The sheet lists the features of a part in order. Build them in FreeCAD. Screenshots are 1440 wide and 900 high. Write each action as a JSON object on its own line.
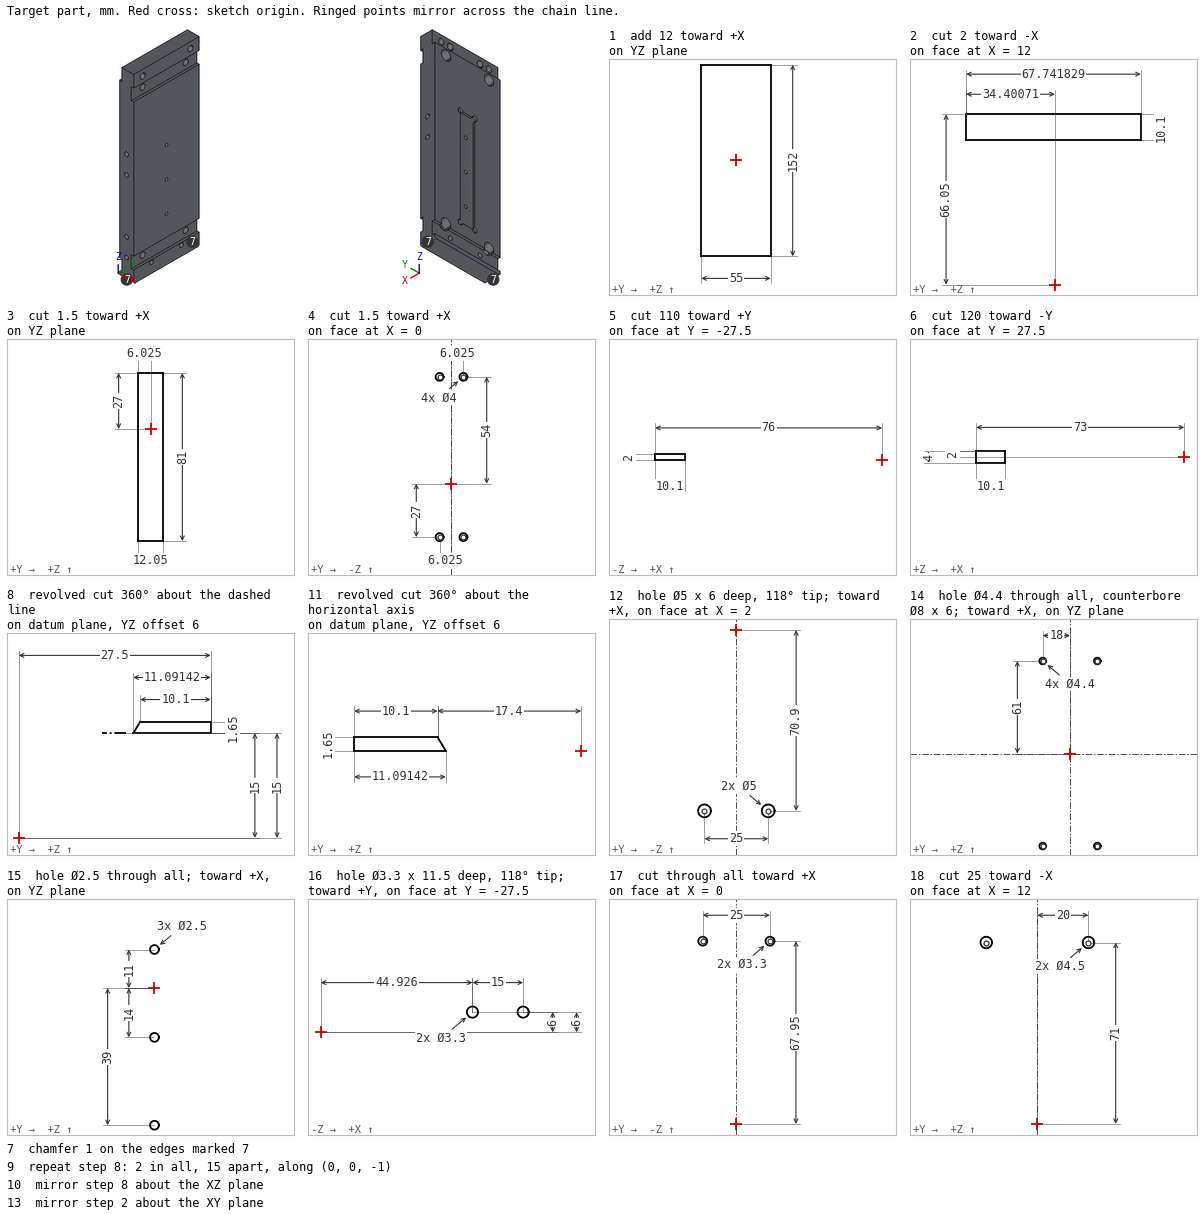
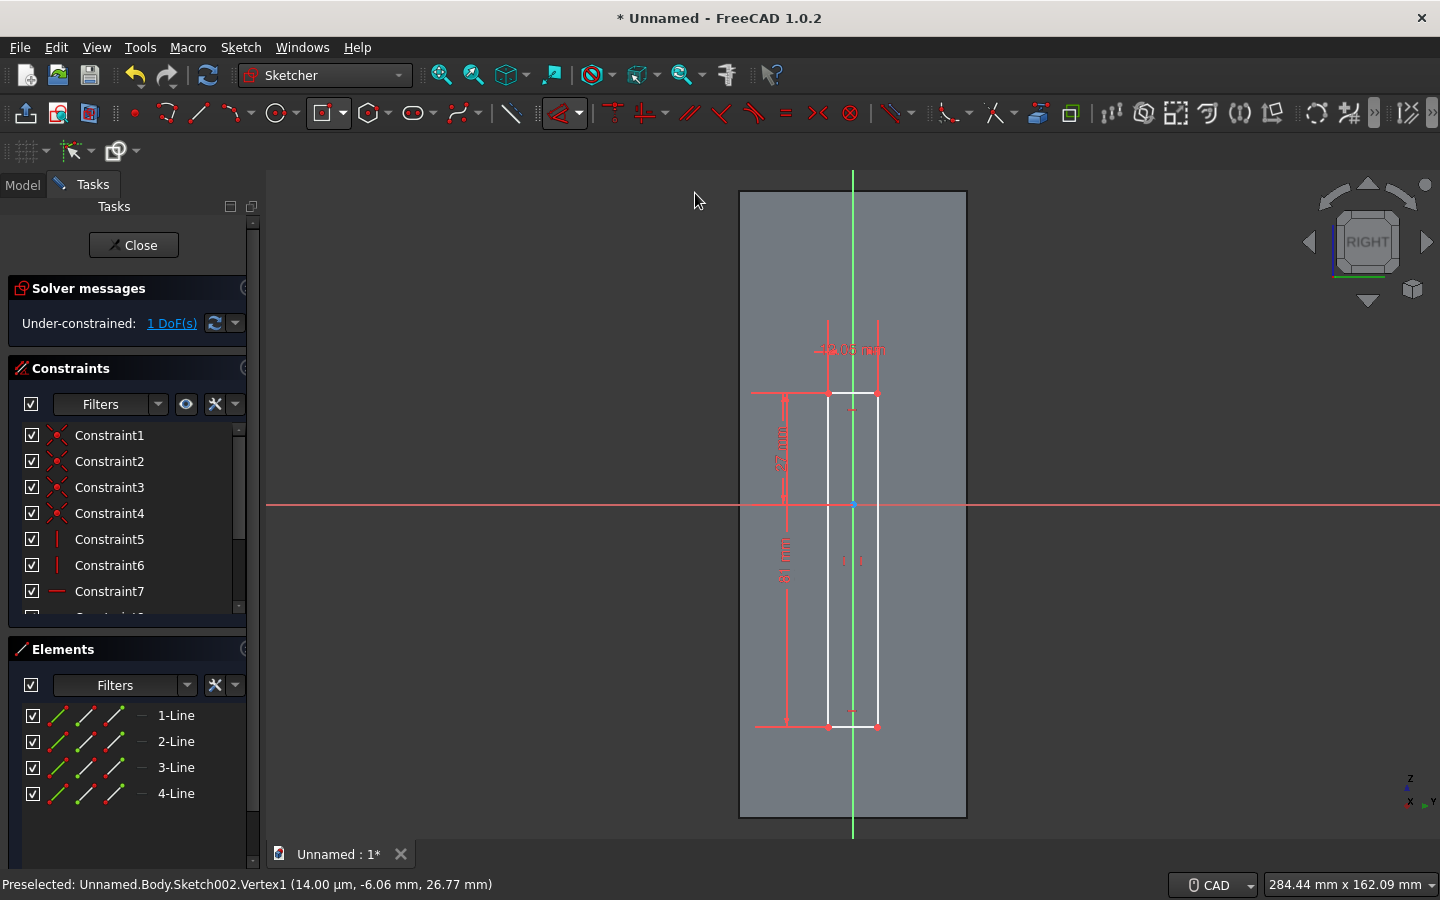
{"action": "scroll", "coordinate": [828, 393], "scroll_direction": "up", "scroll_amount": 3}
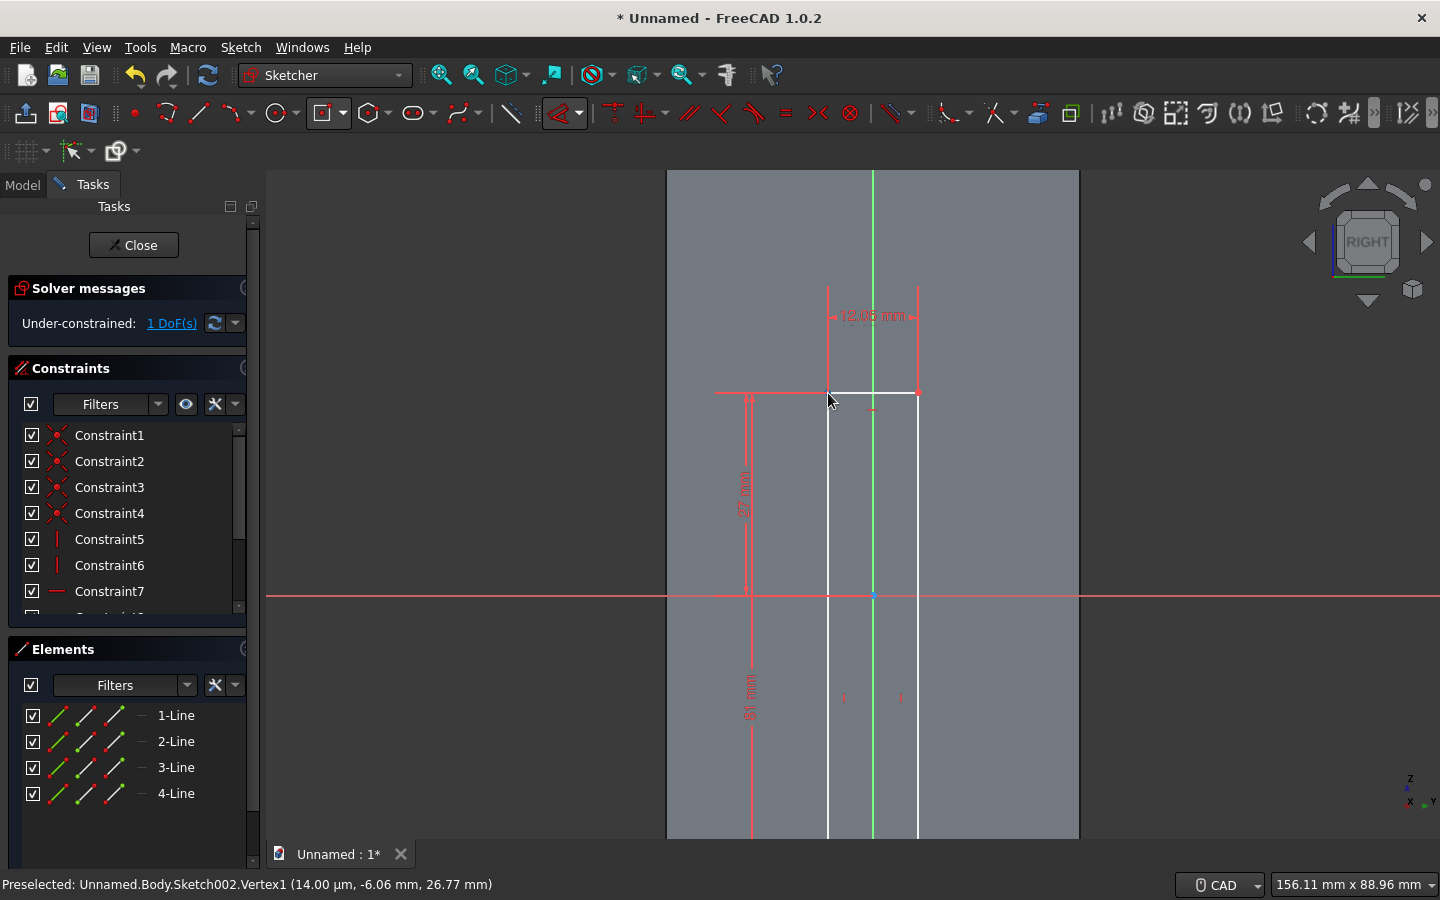
{"action": "left_click", "coordinate": [828, 393]}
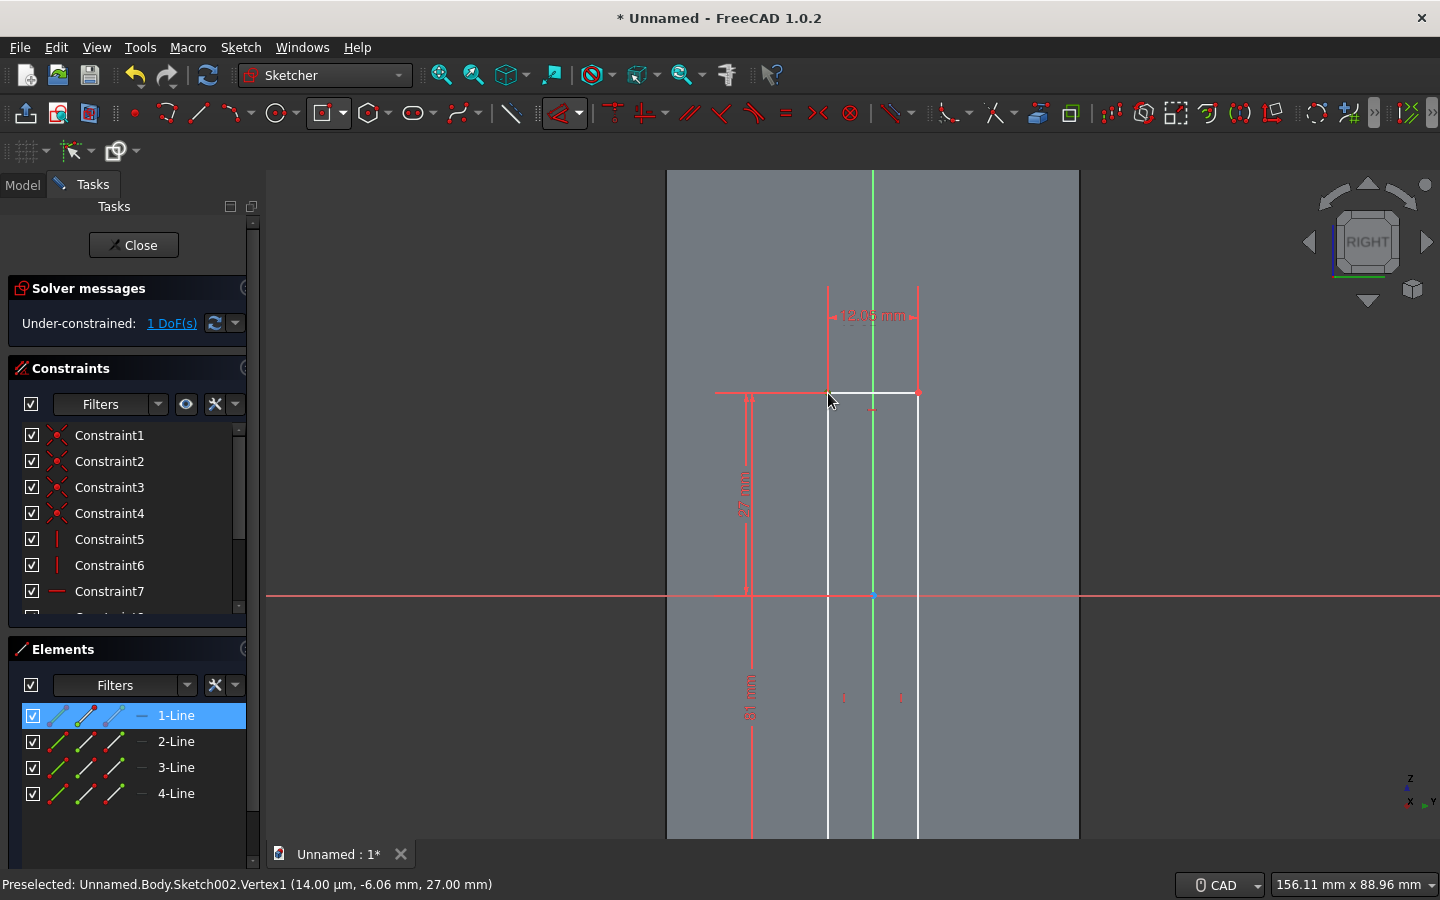
{"action": "key", "text": "l"}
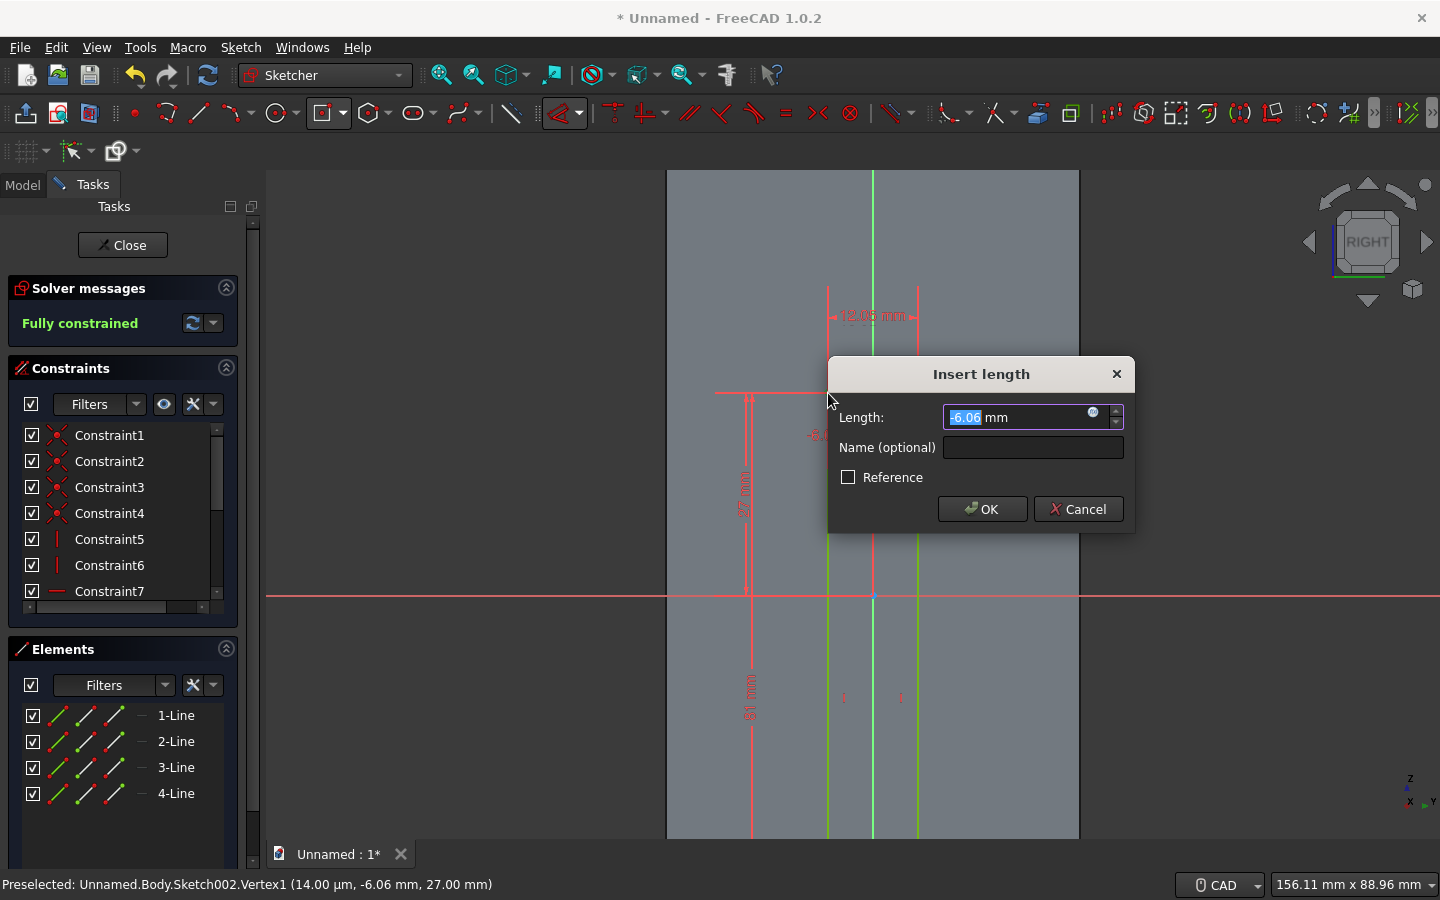
{"action": "type", "text": "-6.025"}
{"action": "key", "text": "Return"}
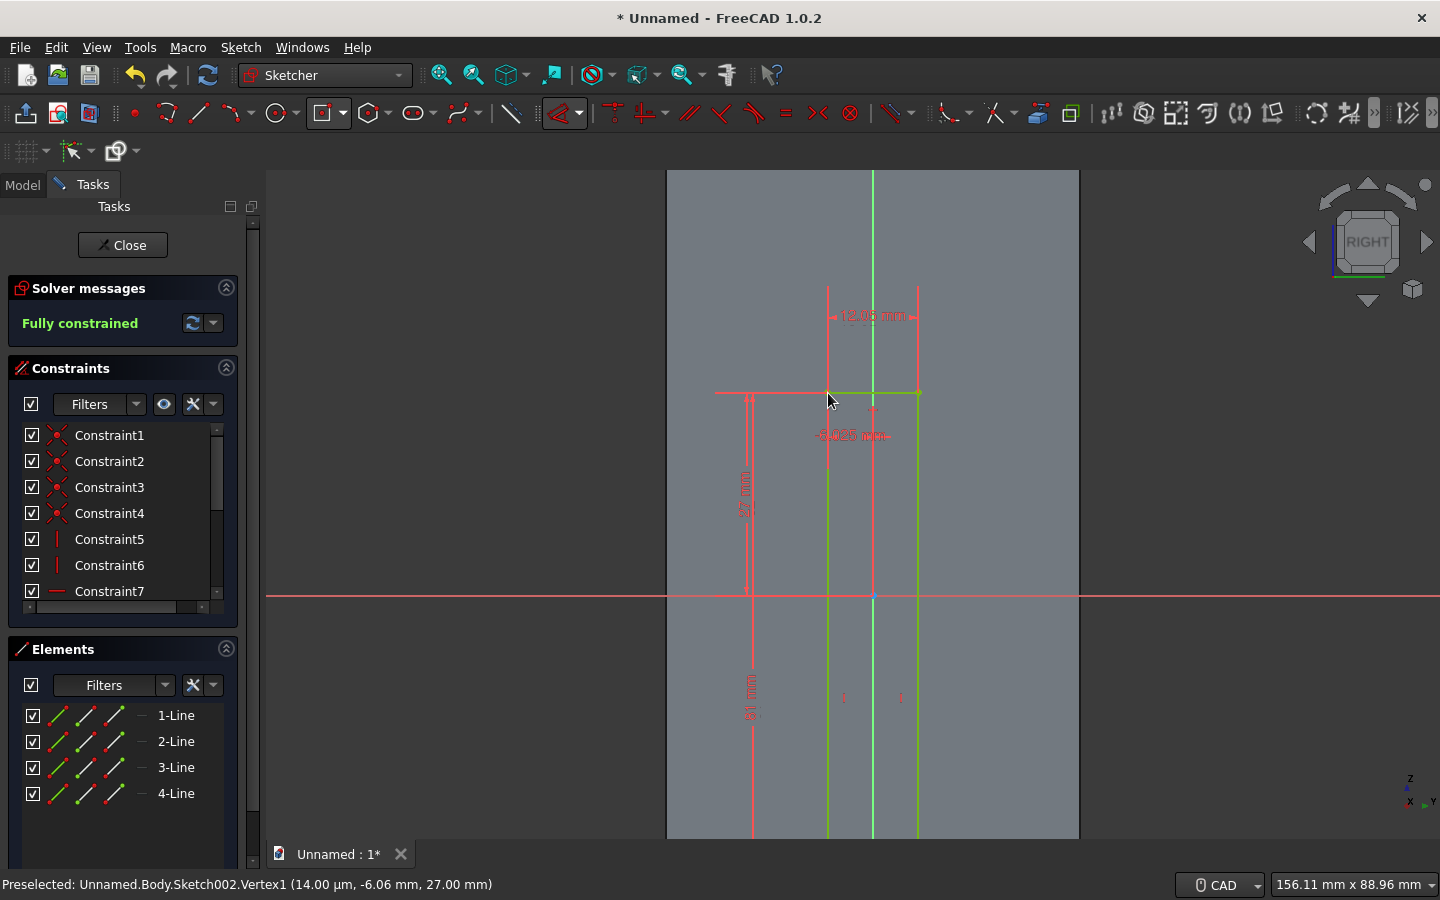
{"action": "left_click", "coordinate": [123, 245]}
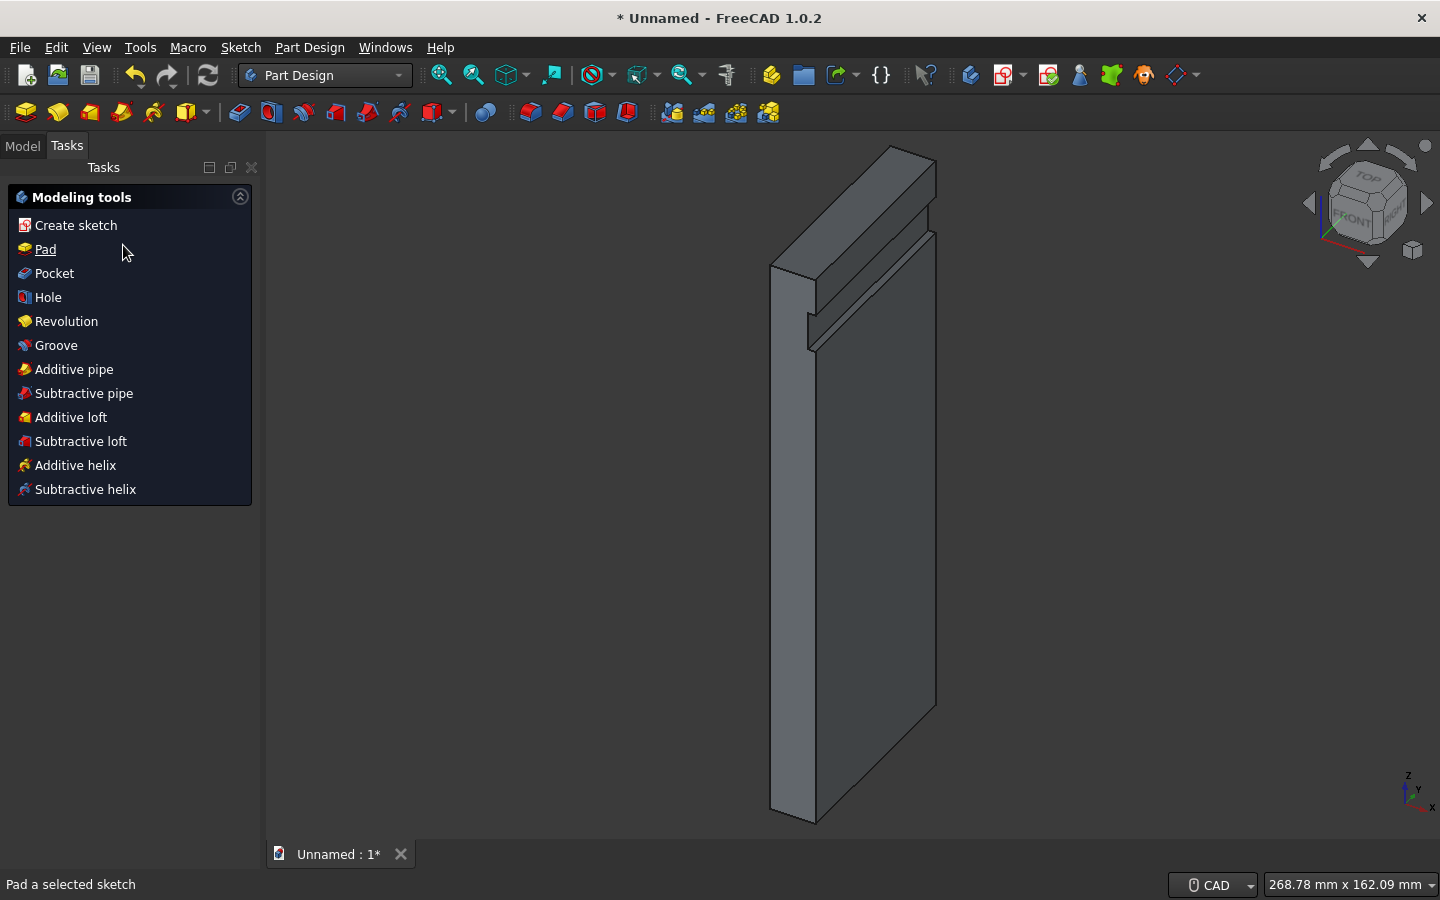
{"action": "left_click", "coordinate": [240, 112]}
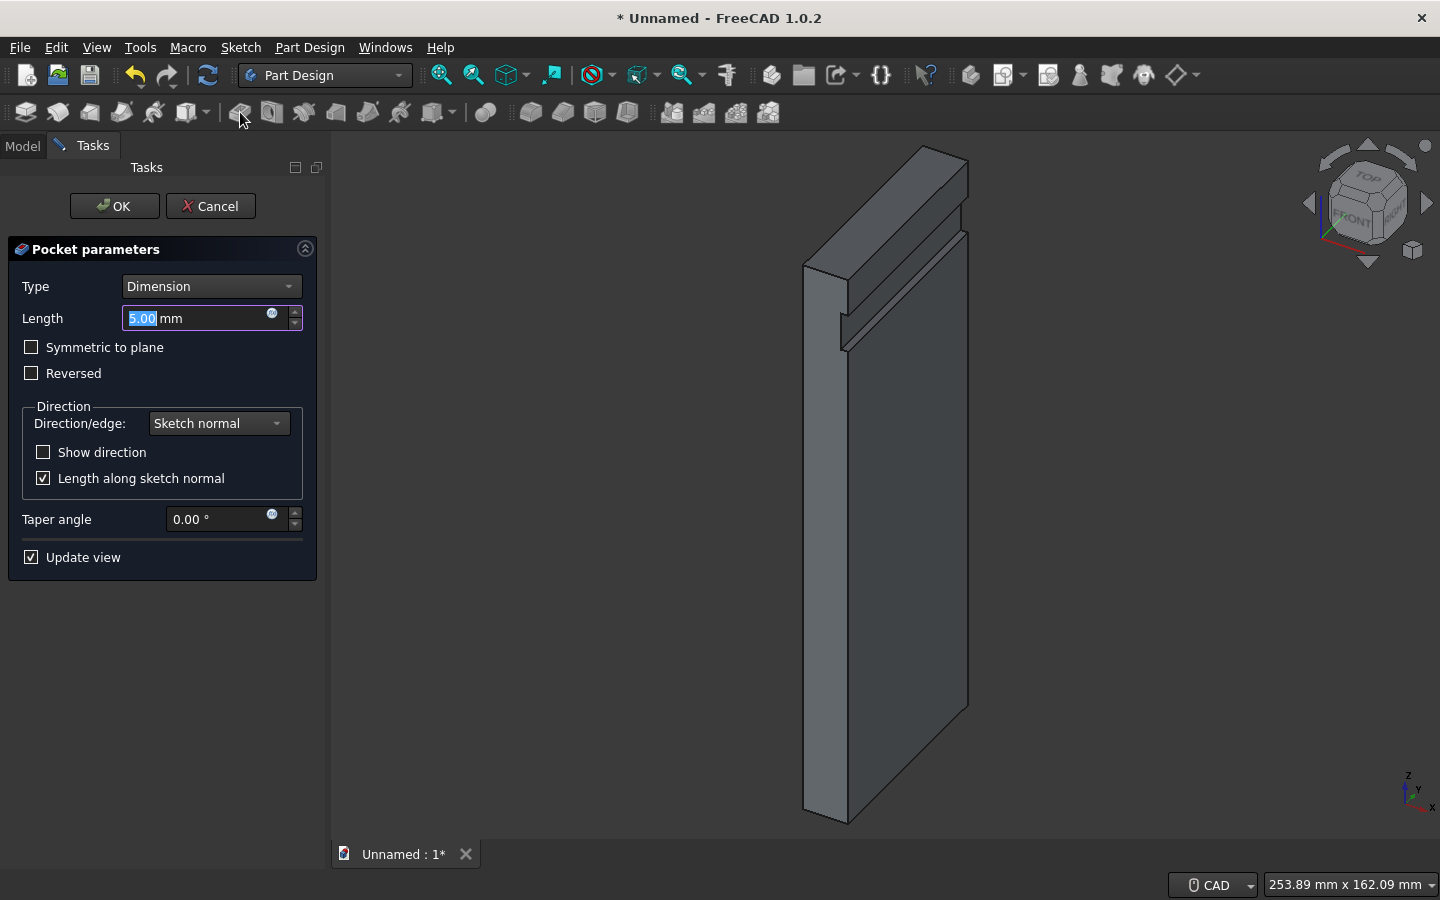
{"action": "type", "text": "1.5"}
{"action": "key", "text": "Tab"}